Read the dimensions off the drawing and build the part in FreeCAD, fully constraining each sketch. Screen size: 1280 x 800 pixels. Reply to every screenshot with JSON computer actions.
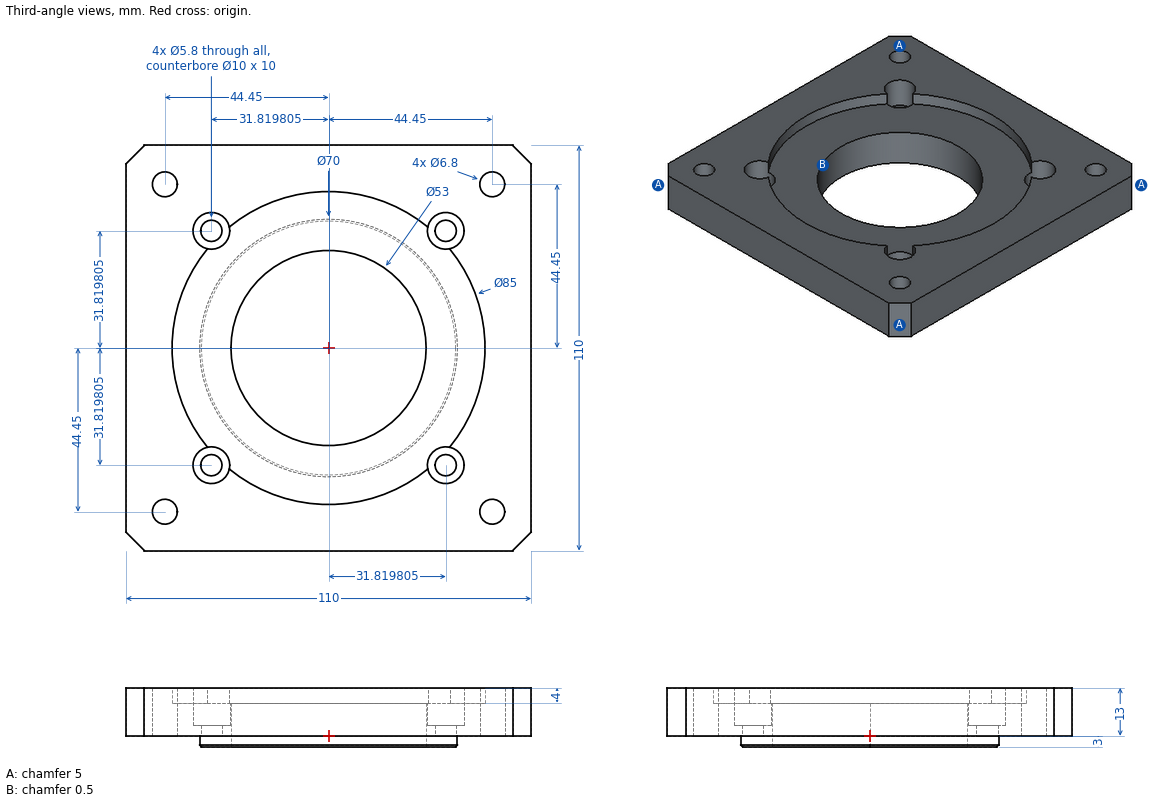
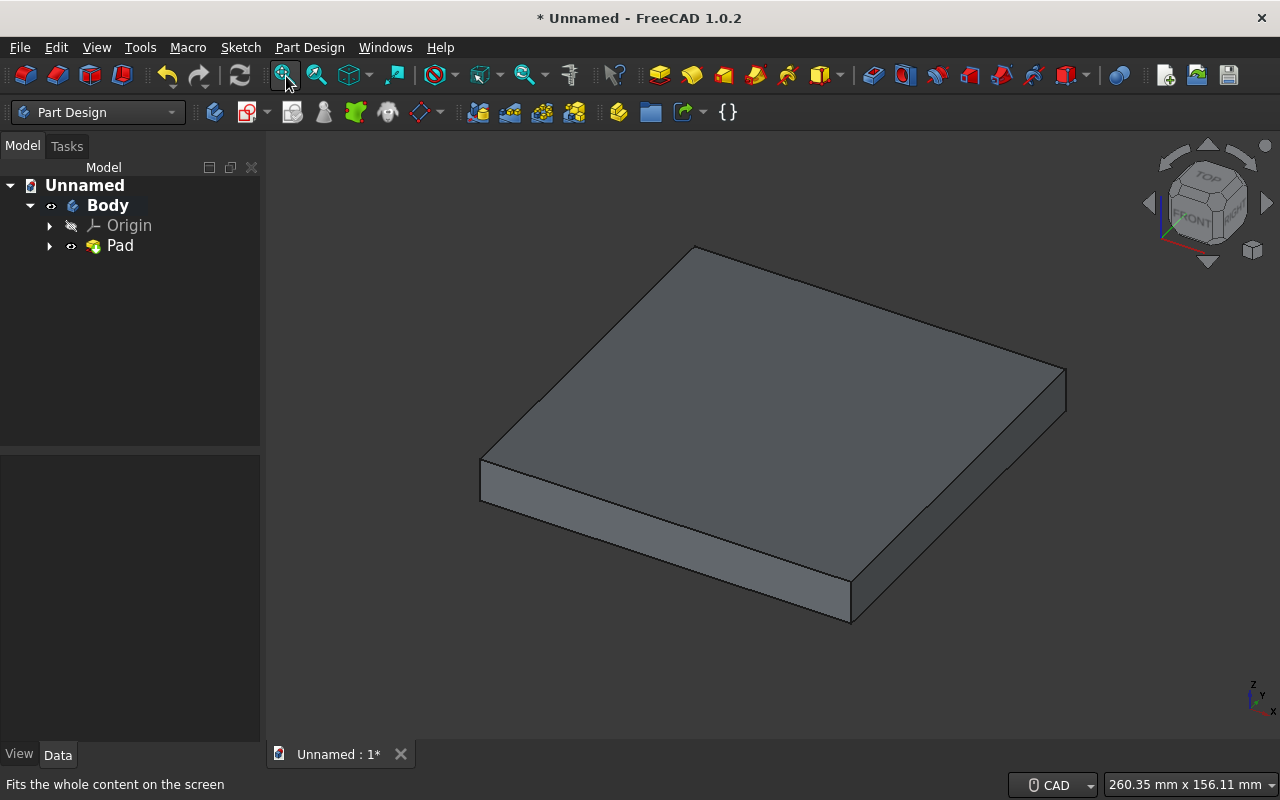
{"action": "left_click", "coordinate": [773, 413]}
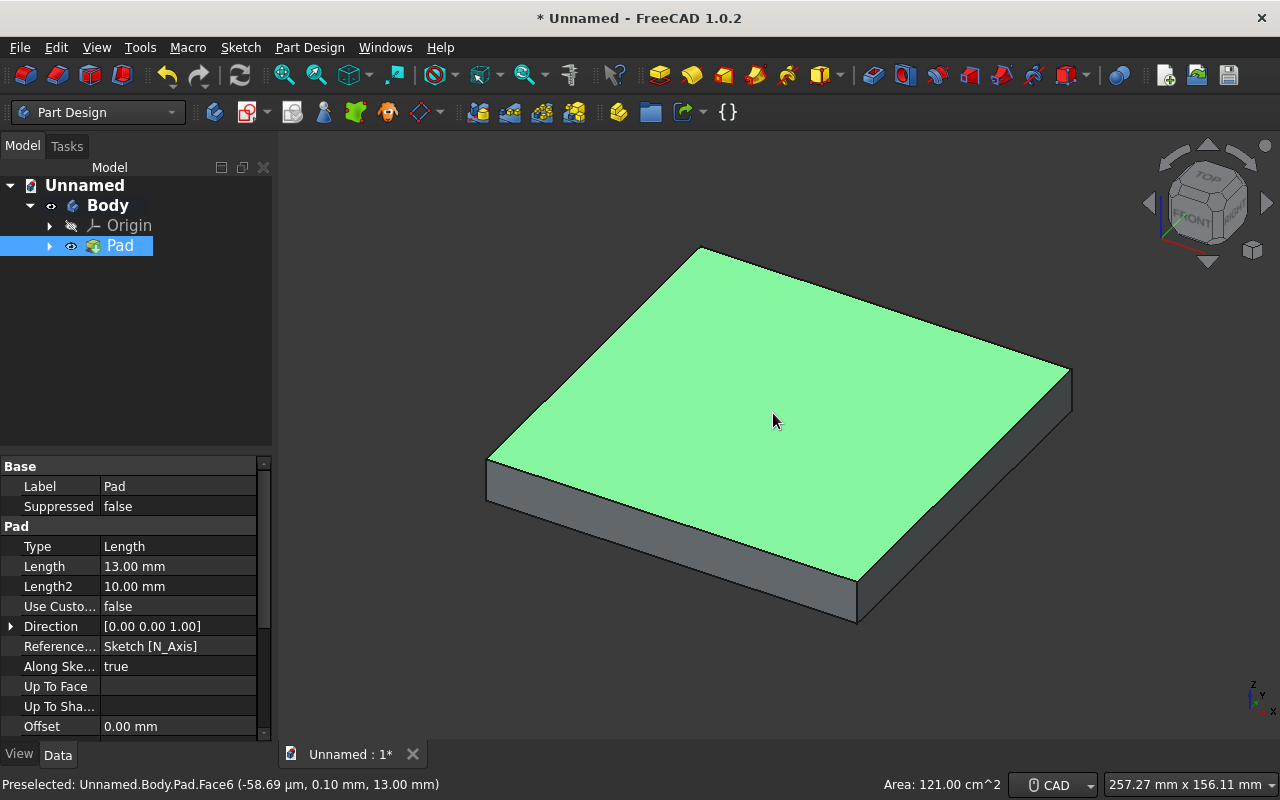
{"action": "left_click", "coordinate": [248, 112]}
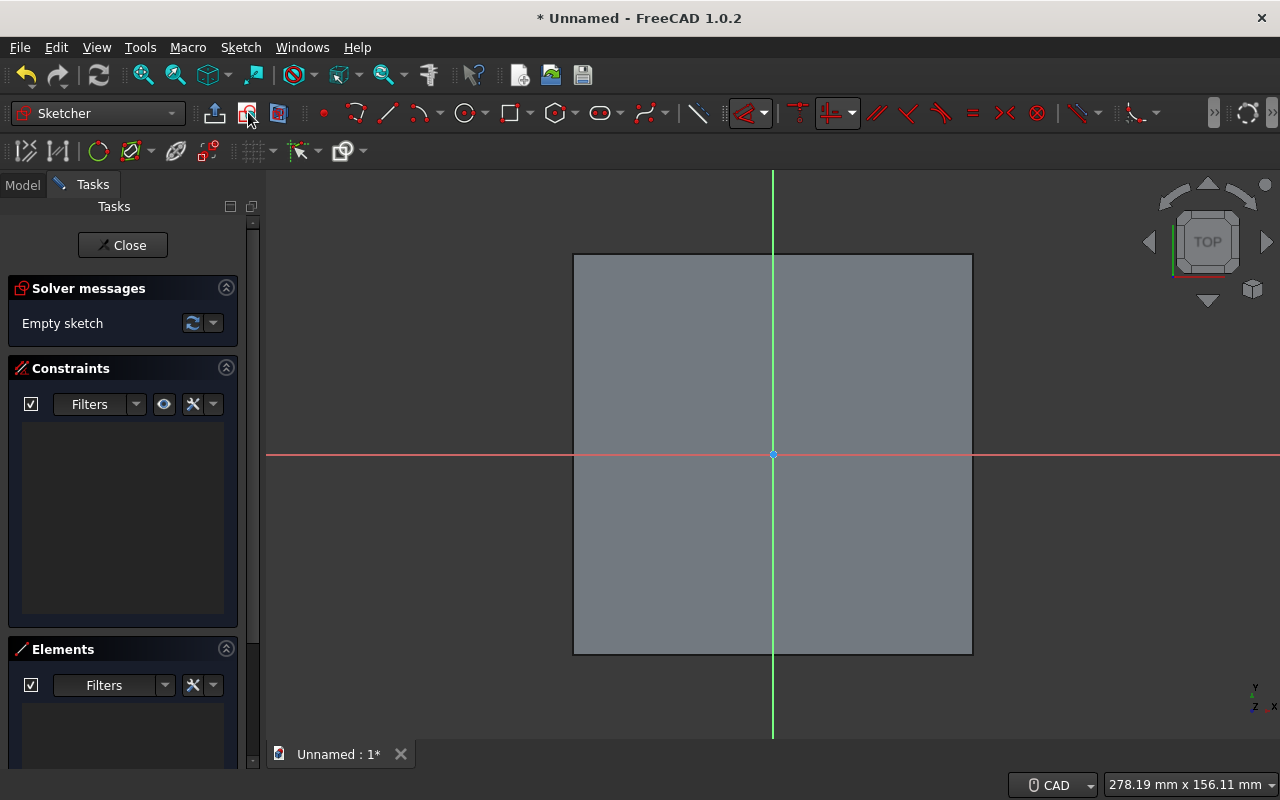
{"action": "key", "text": "g c"}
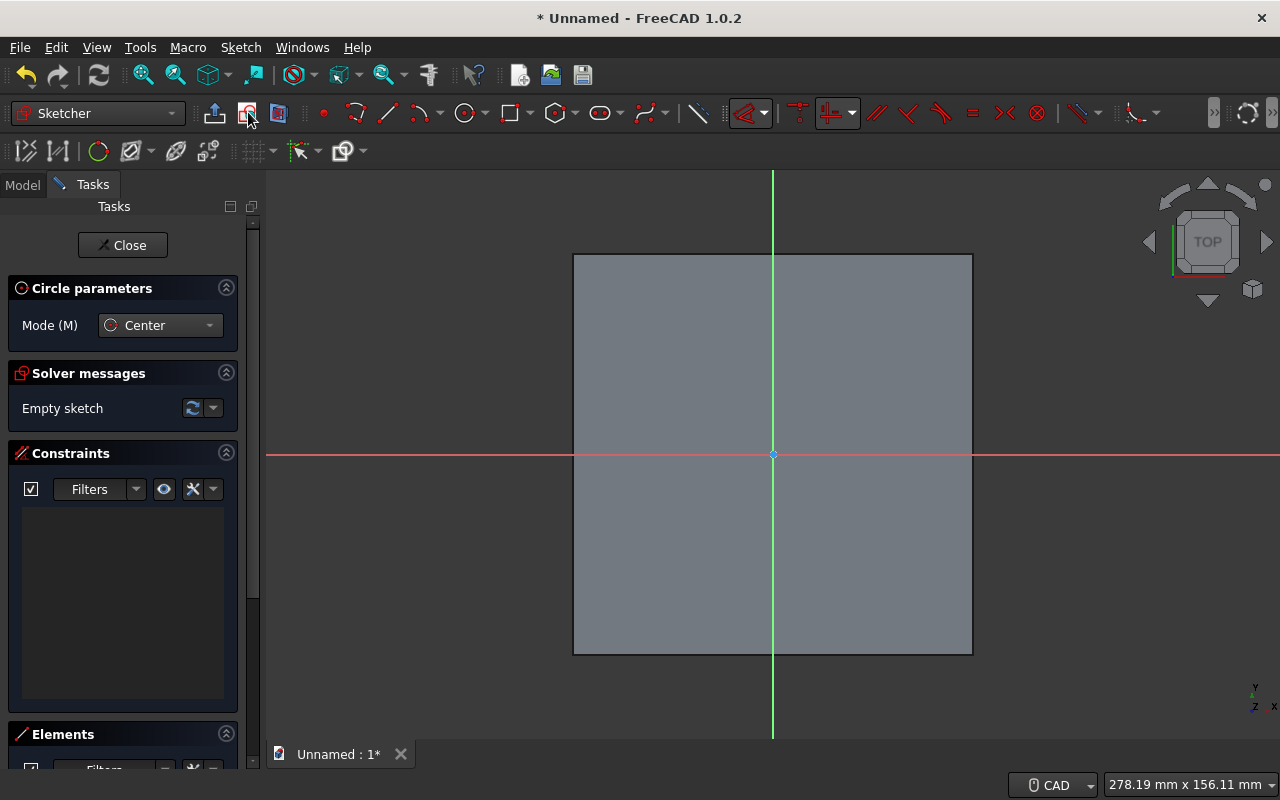
{"action": "left_click", "coordinate": [773, 454]}
{"action": "left_click", "coordinate": [883, 345]}
{"action": "key", "text": "Escape"}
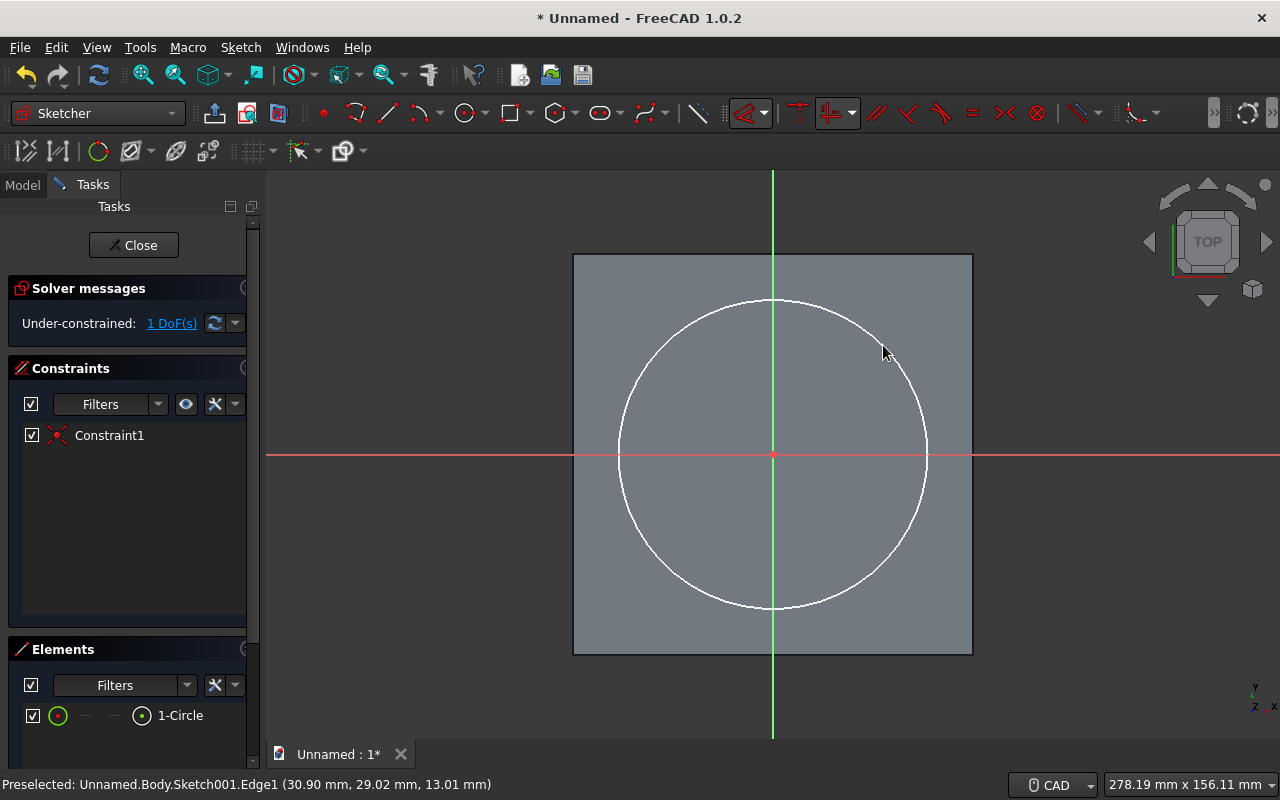
{"action": "left_click", "coordinate": [882, 345]}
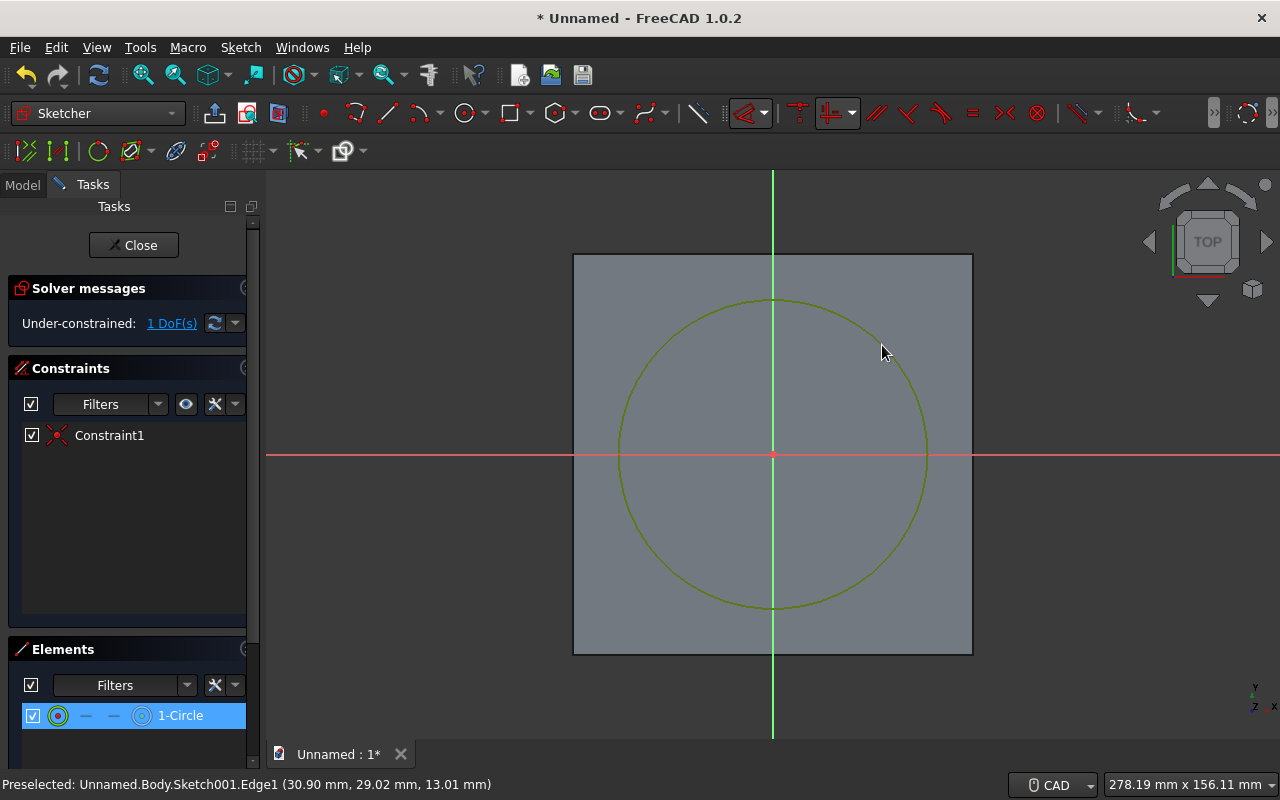
{"action": "key", "text": "k o"}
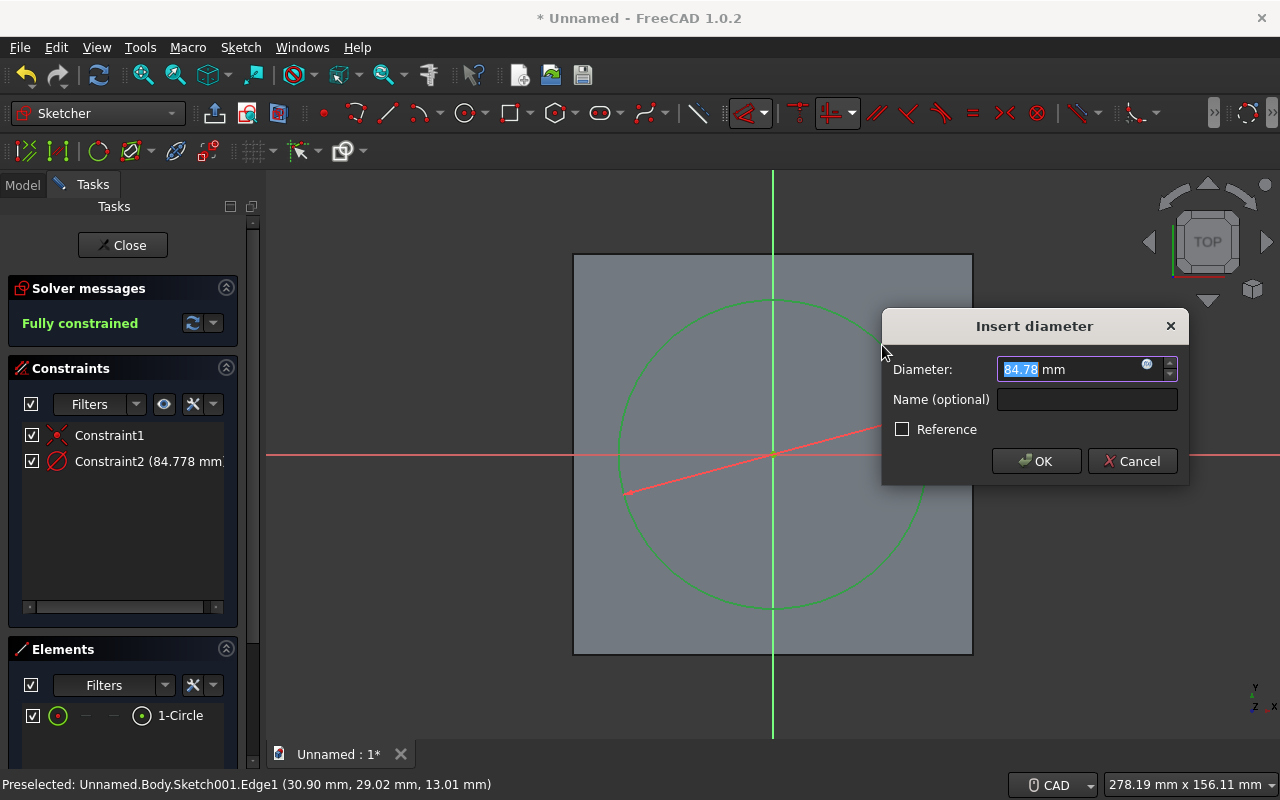
{"action": "type", "text": "85"}
{"action": "key", "text": "Return"}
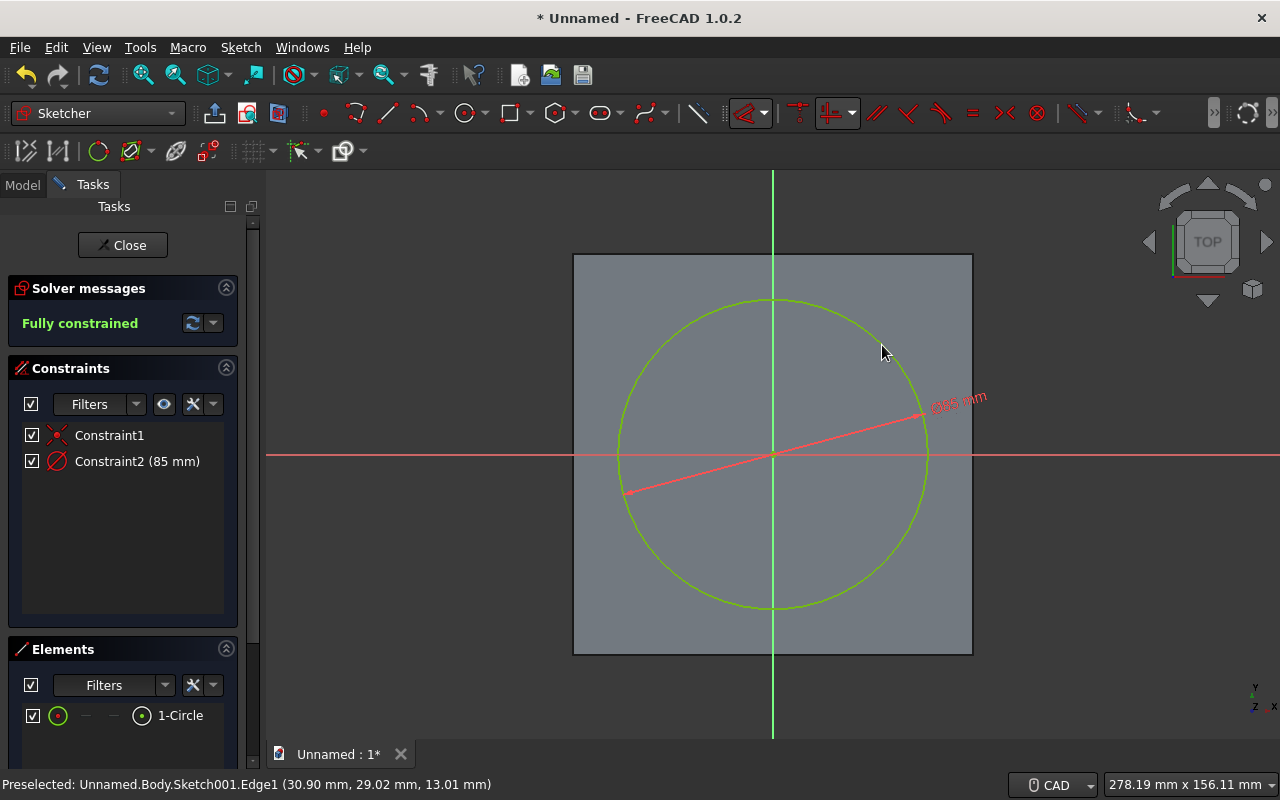
{"action": "left_click", "coordinate": [123, 245]}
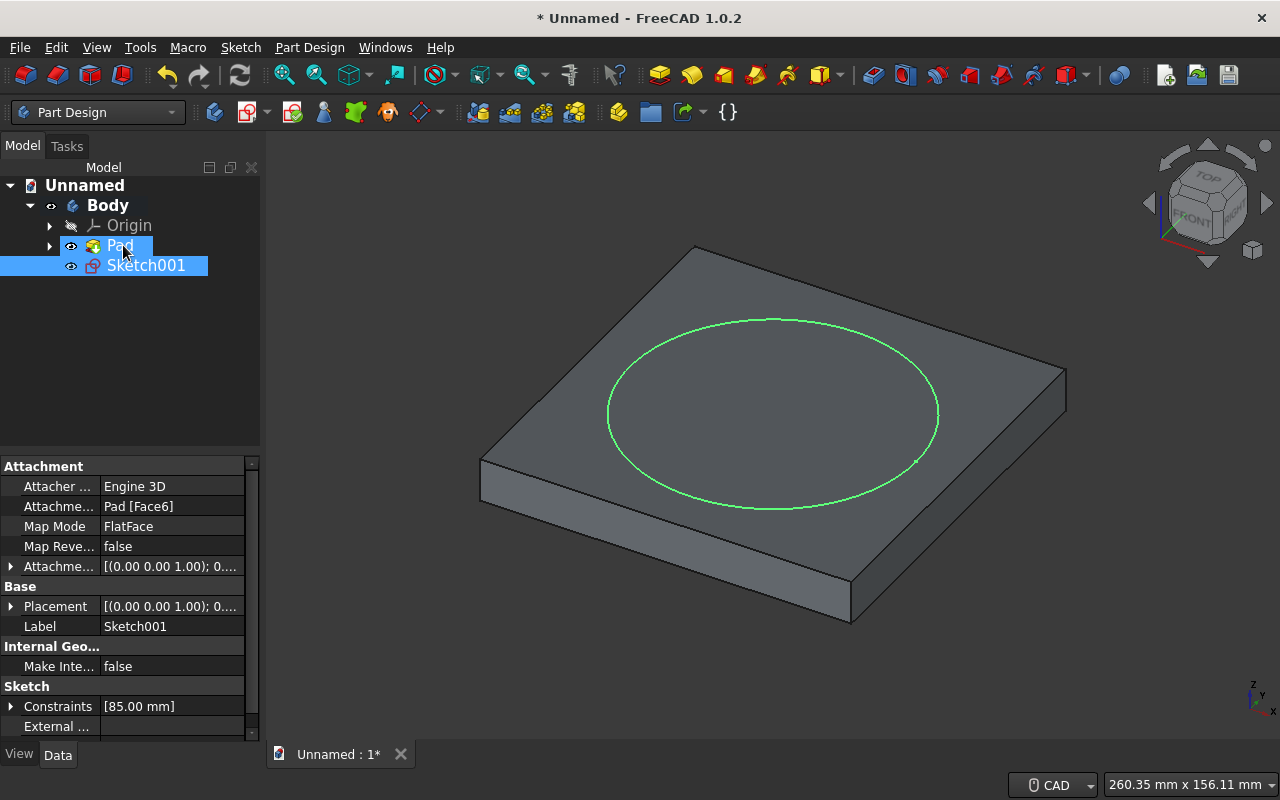
{"action": "left_click", "coordinate": [874, 76]}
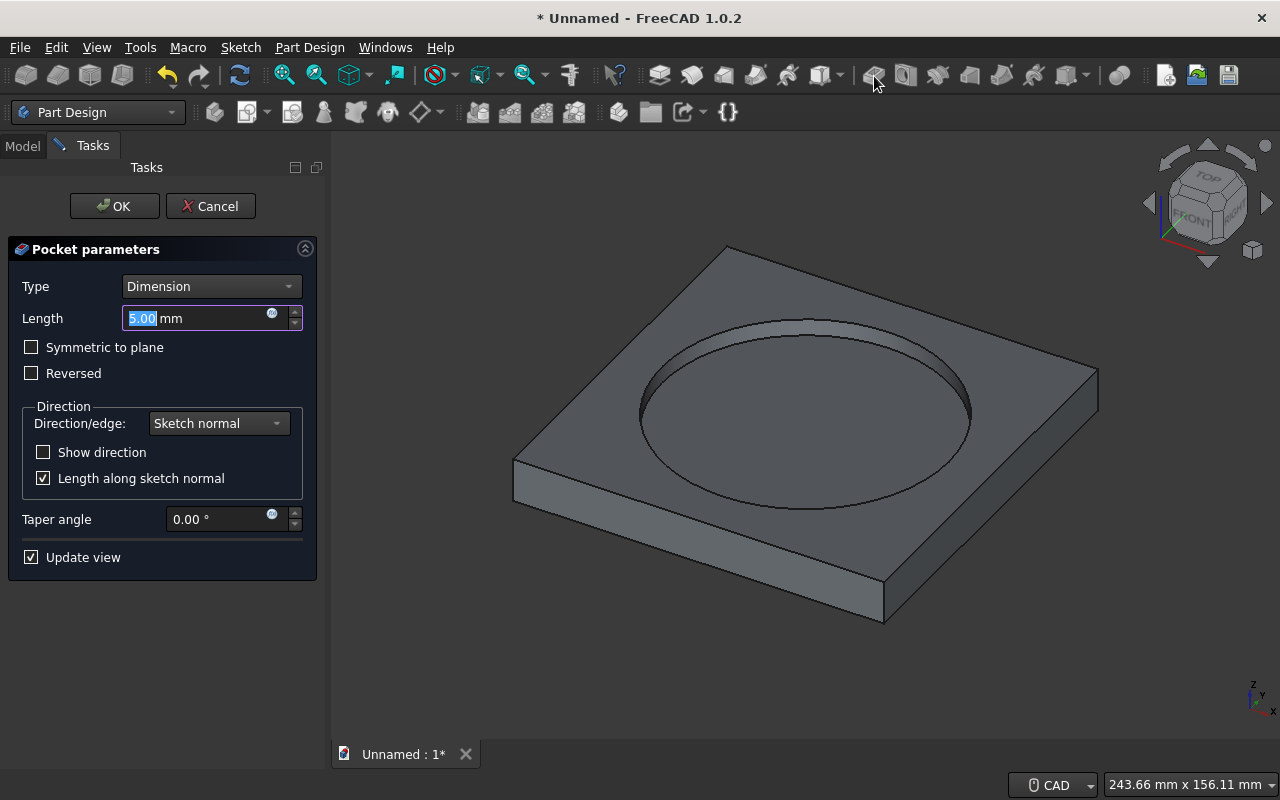
{"action": "type", "text": "4"}
{"action": "key", "text": "Tab"}